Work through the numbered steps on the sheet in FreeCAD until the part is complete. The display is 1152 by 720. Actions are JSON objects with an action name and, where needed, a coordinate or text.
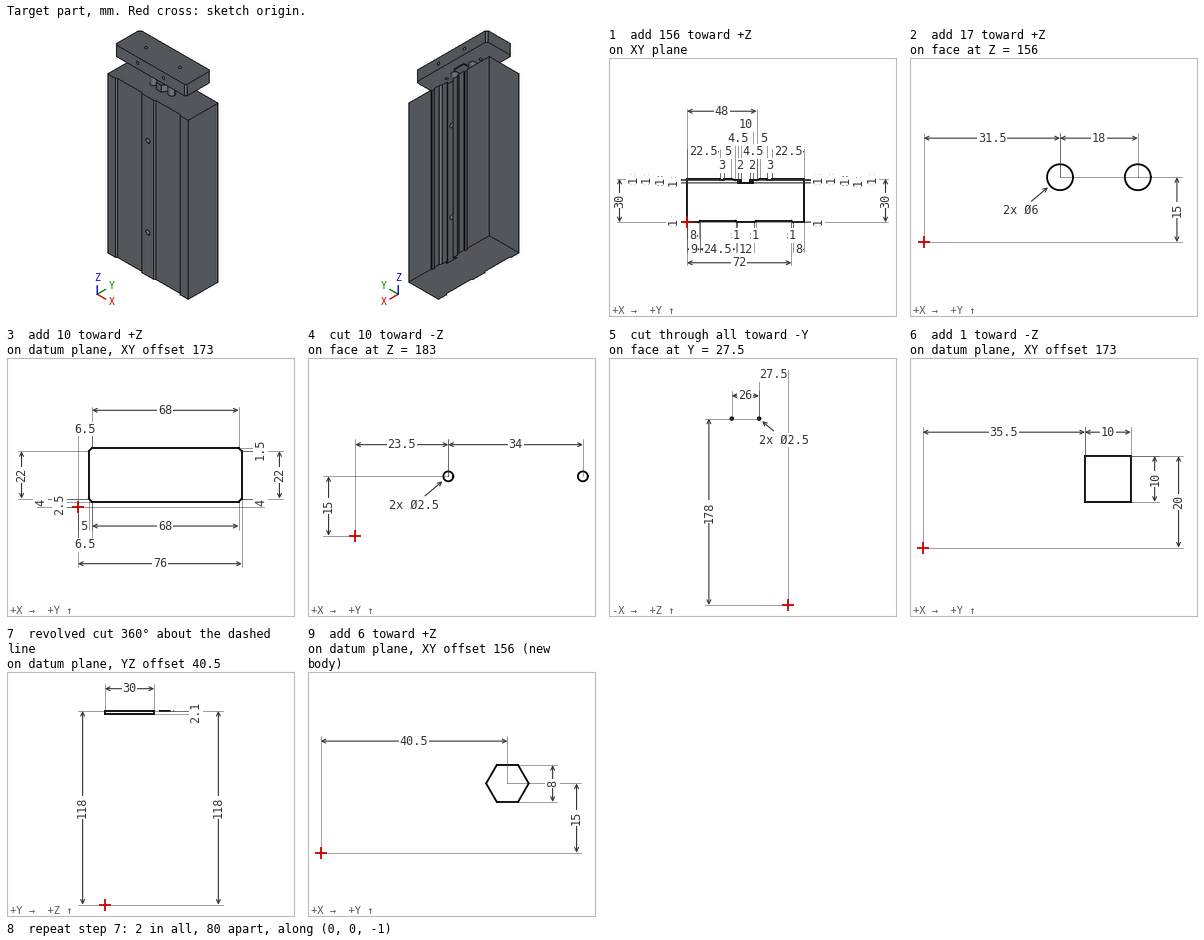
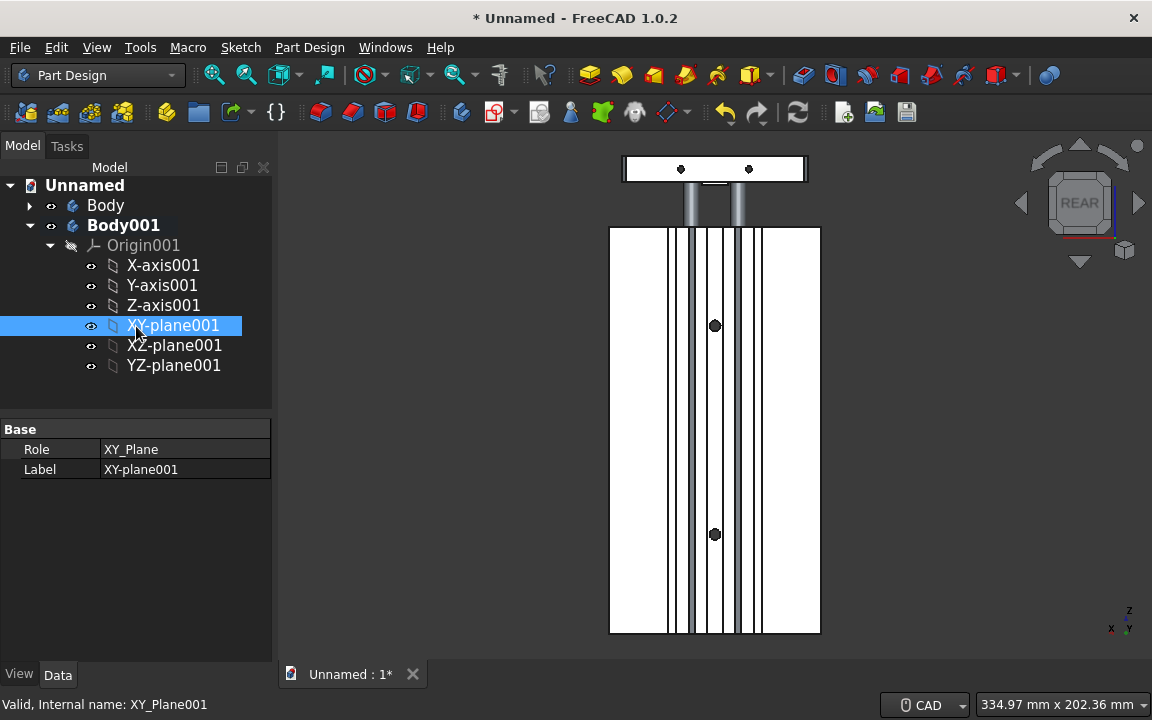
{"action": "left_click", "coordinate": [668, 112]}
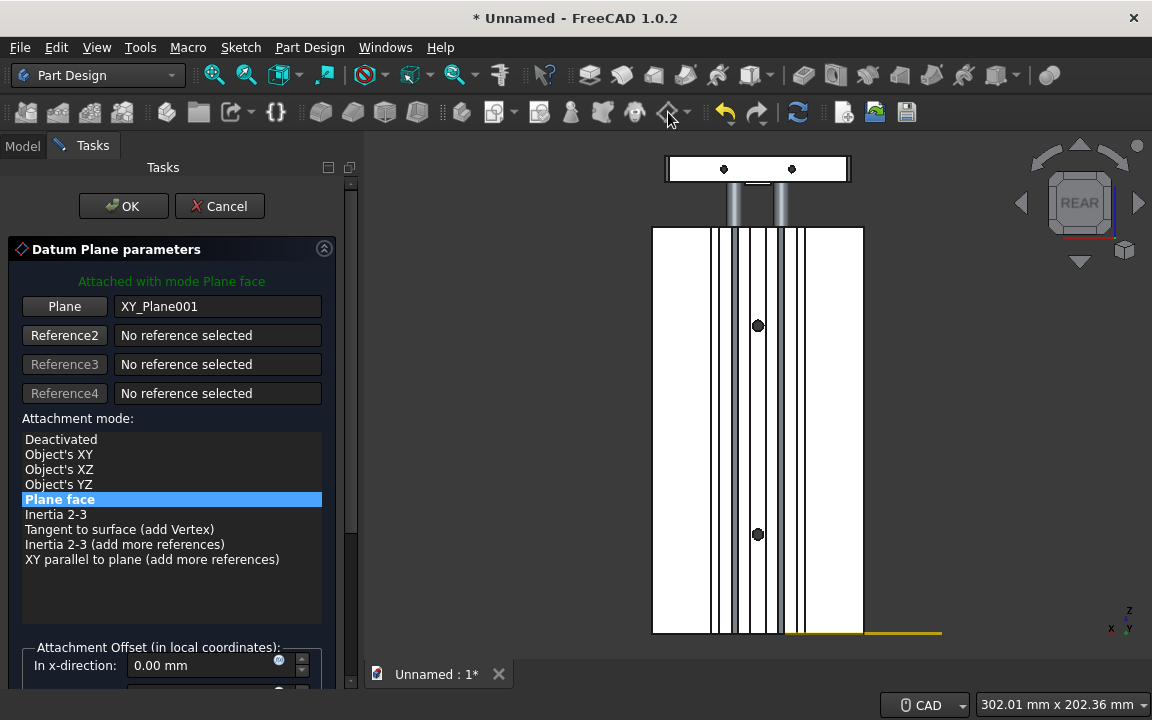
{"action": "scroll", "coordinate": [351, 432], "scroll_direction": "down", "scroll_amount": 2}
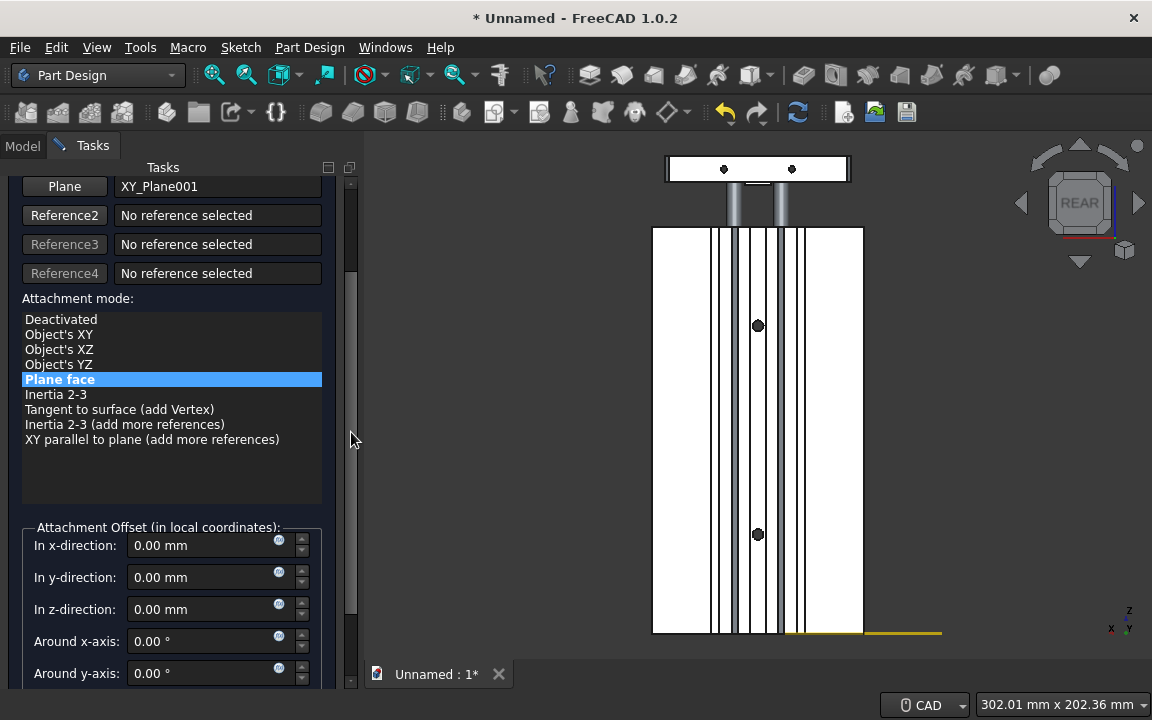
{"action": "triple_click", "coordinate": [210, 609]}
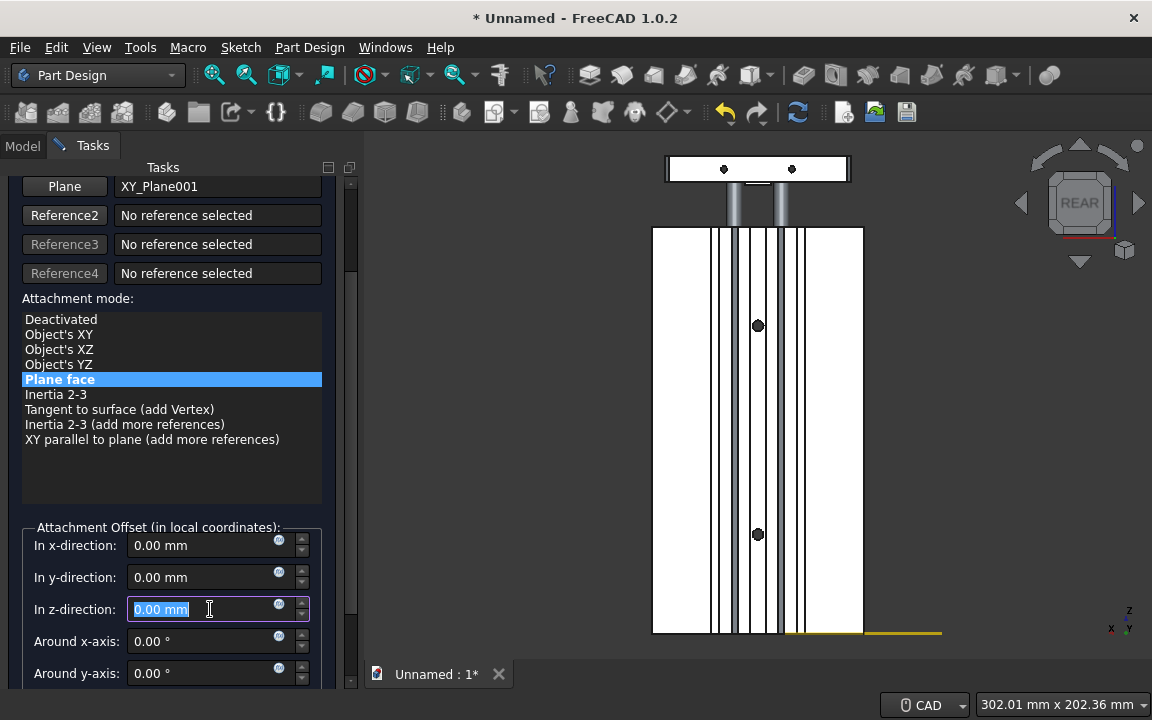
{"action": "type", "text": "156"}
{"action": "key", "text": "Tab"}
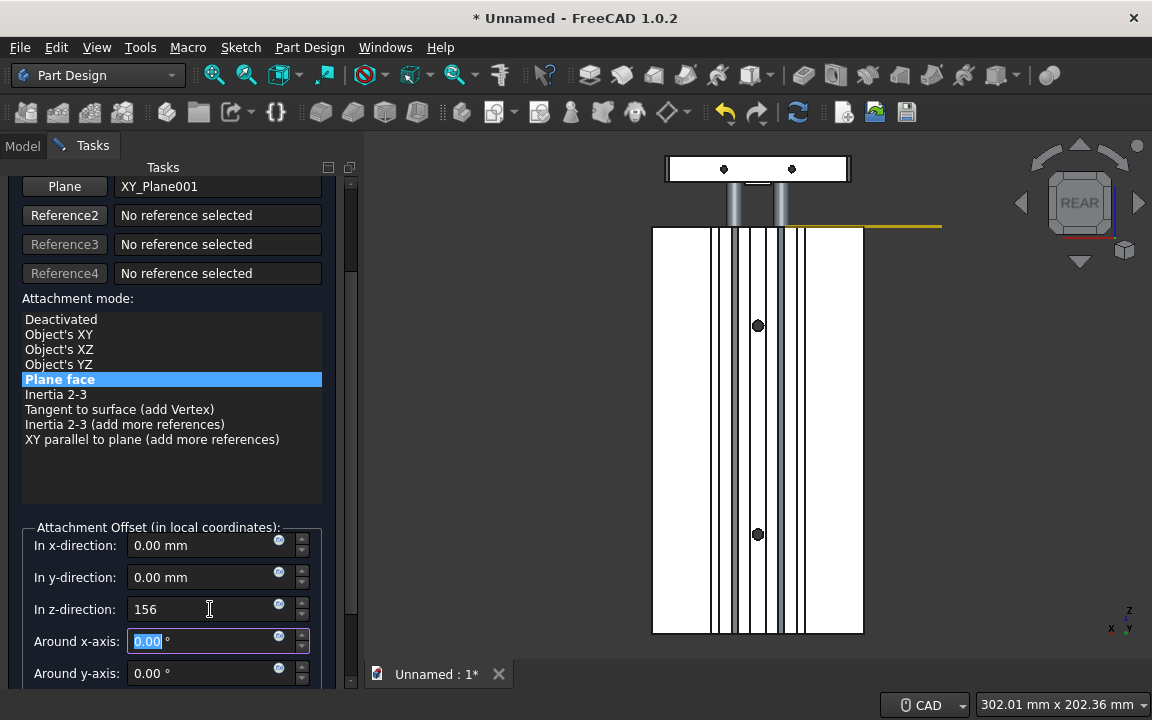
{"action": "scroll", "coordinate": [351, 432], "scroll_direction": "up", "scroll_amount": 3}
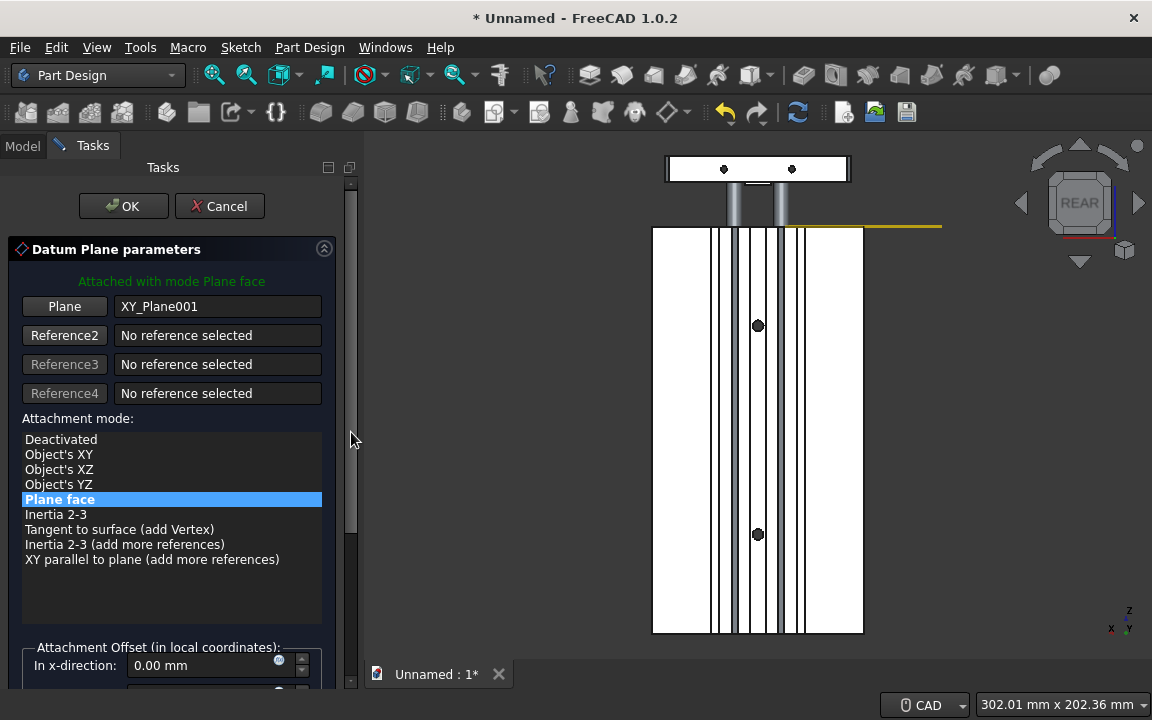
{"action": "left_click", "coordinate": [124, 206]}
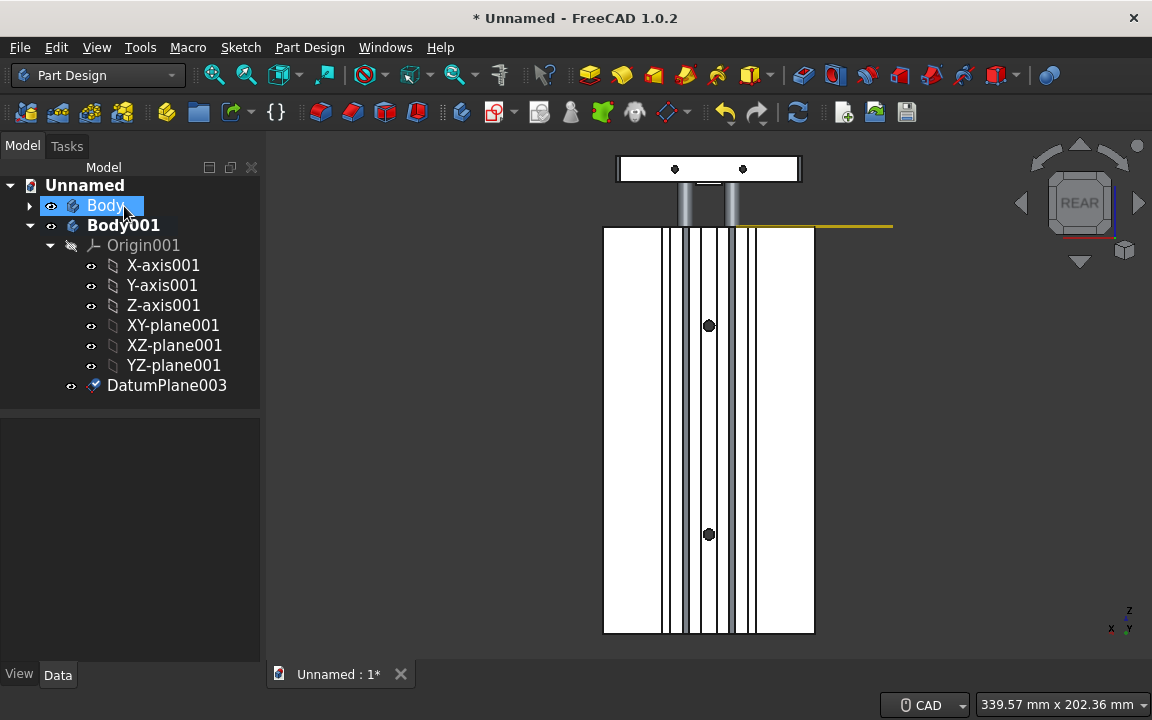
{"action": "left_click", "coordinate": [116, 386]}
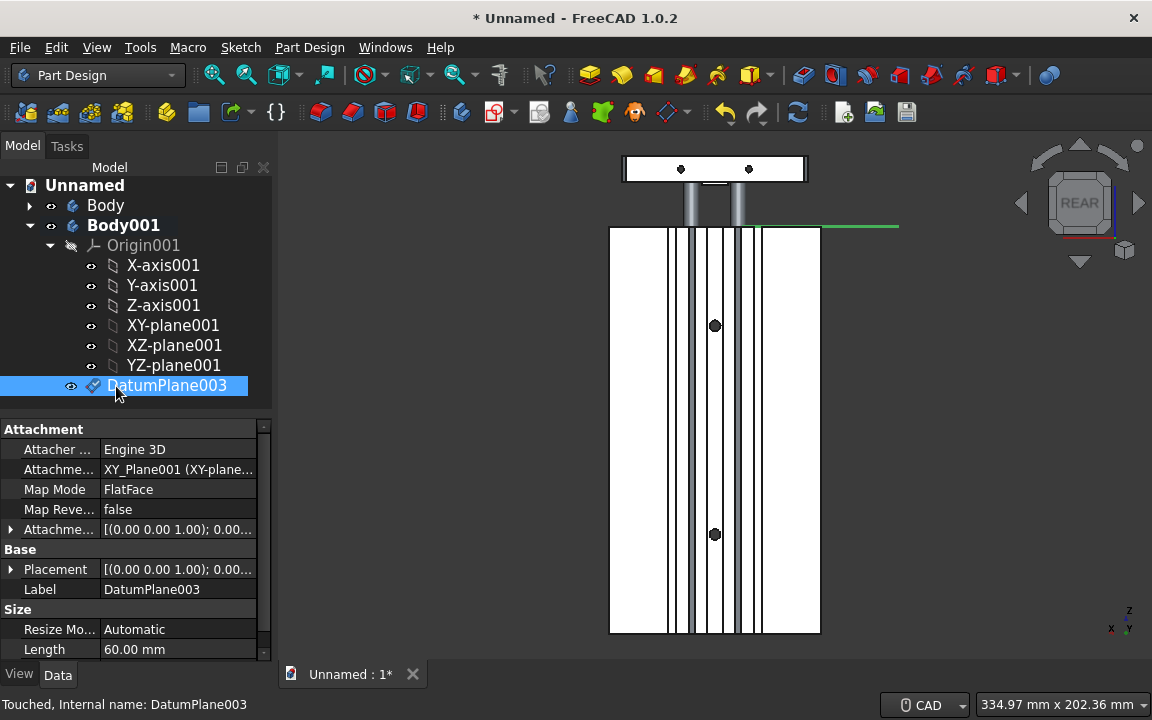
{"action": "left_click", "coordinate": [494, 112]}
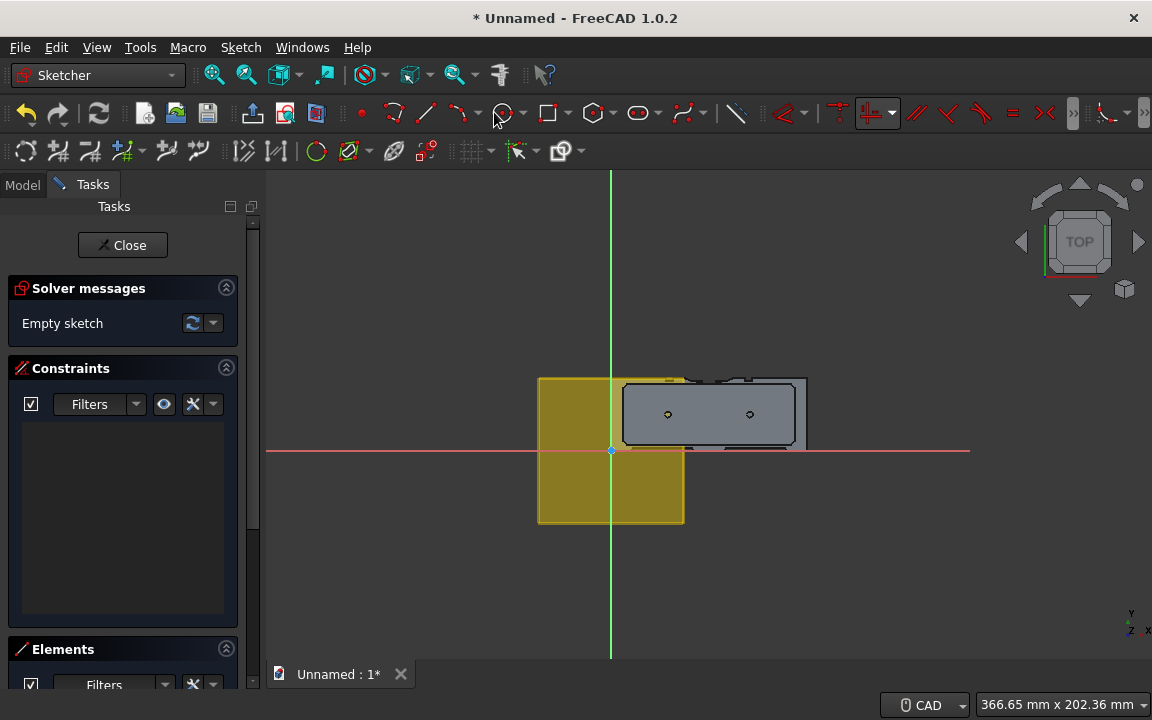
{"action": "scroll", "coordinate": [713, 414], "scroll_direction": "up", "scroll_amount": 14}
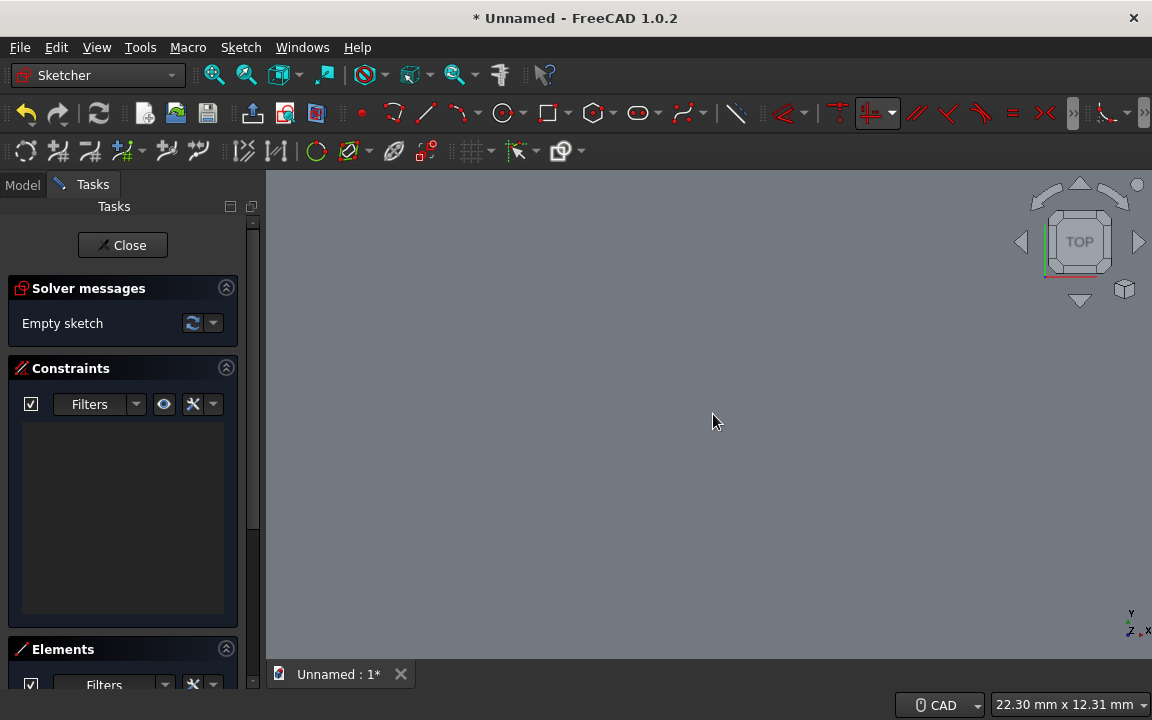
{"action": "key", "text": "g p 6"}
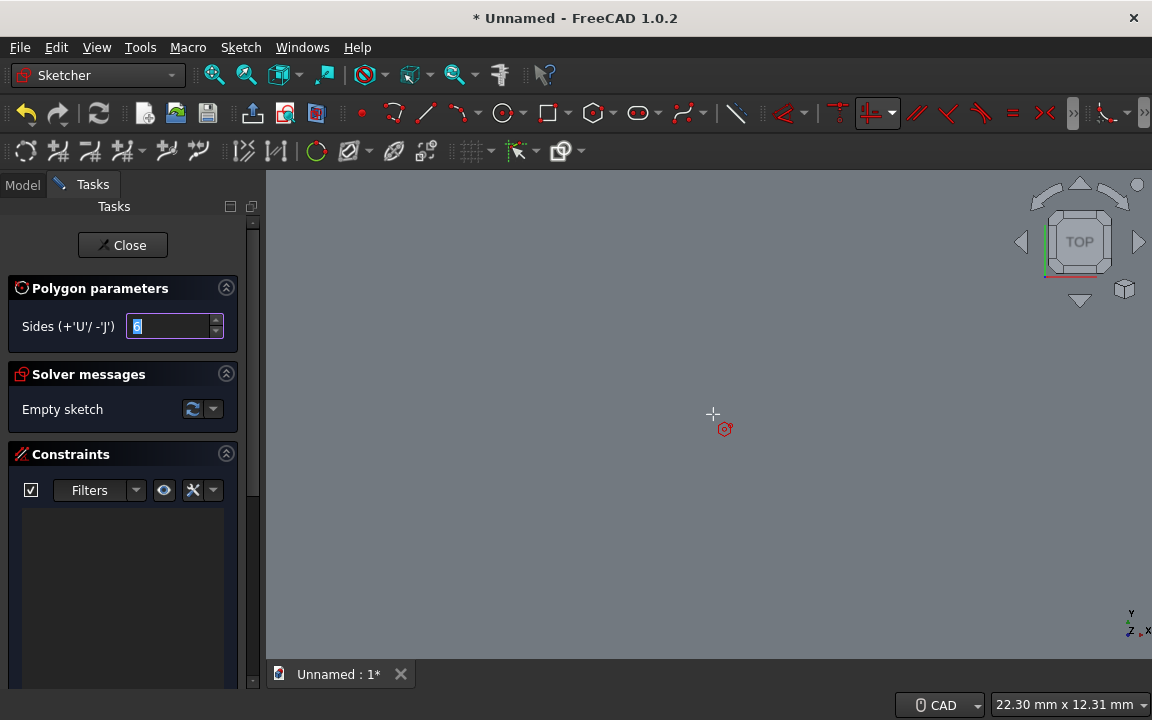
{"action": "left_click", "coordinate": [639, 414]}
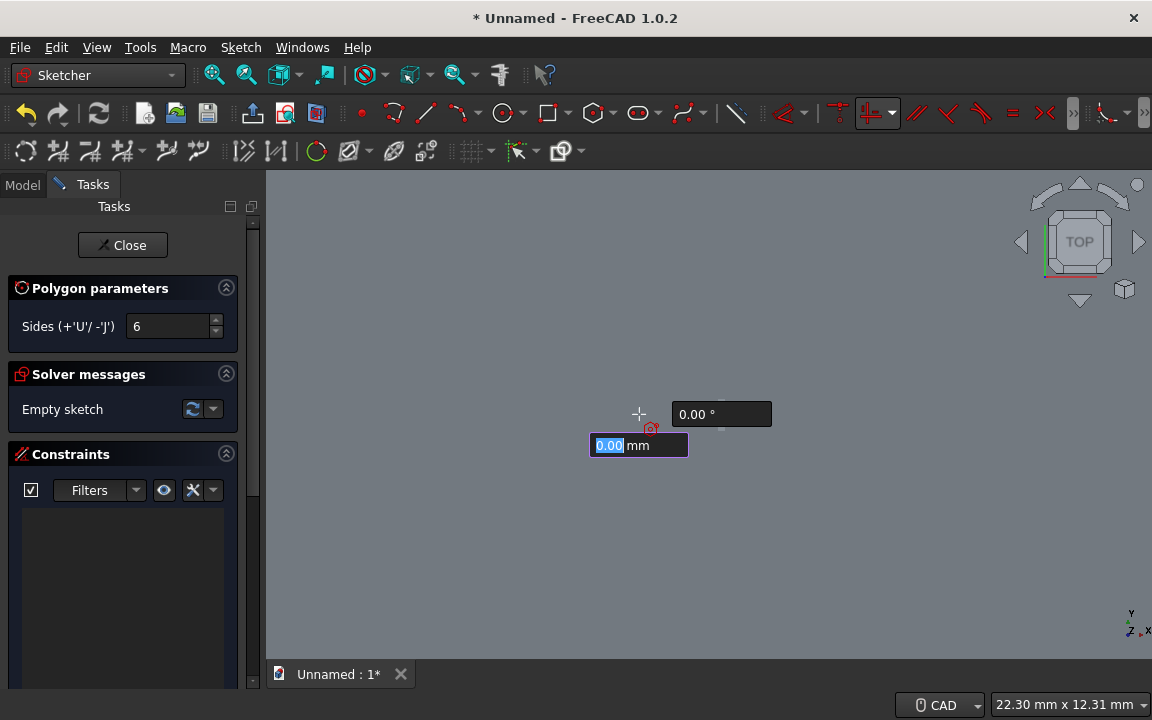
{"action": "left_click", "coordinate": [823, 414]}
{"action": "right_click", "coordinate": [823, 414]}